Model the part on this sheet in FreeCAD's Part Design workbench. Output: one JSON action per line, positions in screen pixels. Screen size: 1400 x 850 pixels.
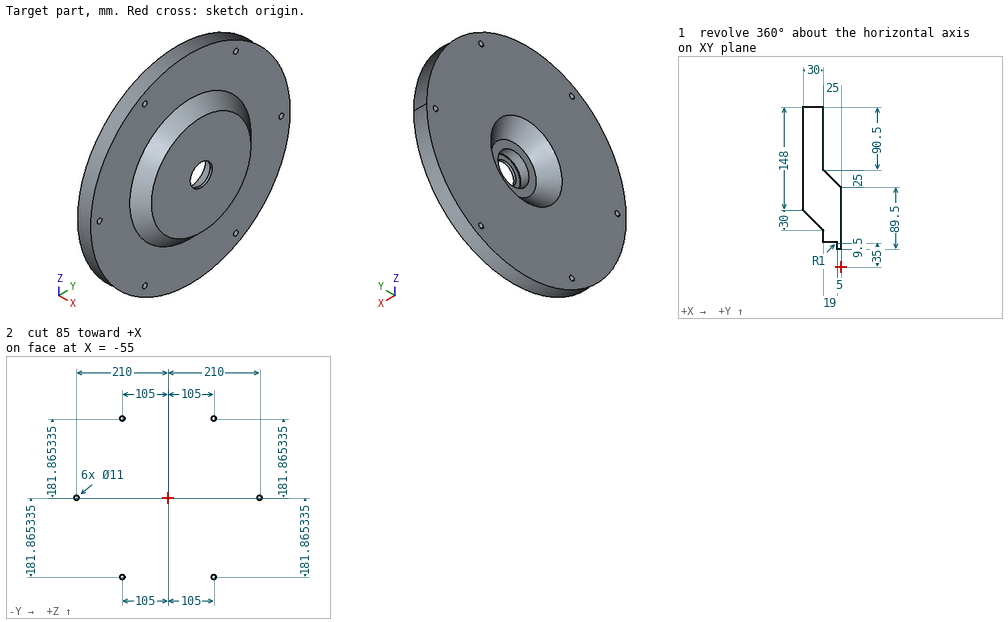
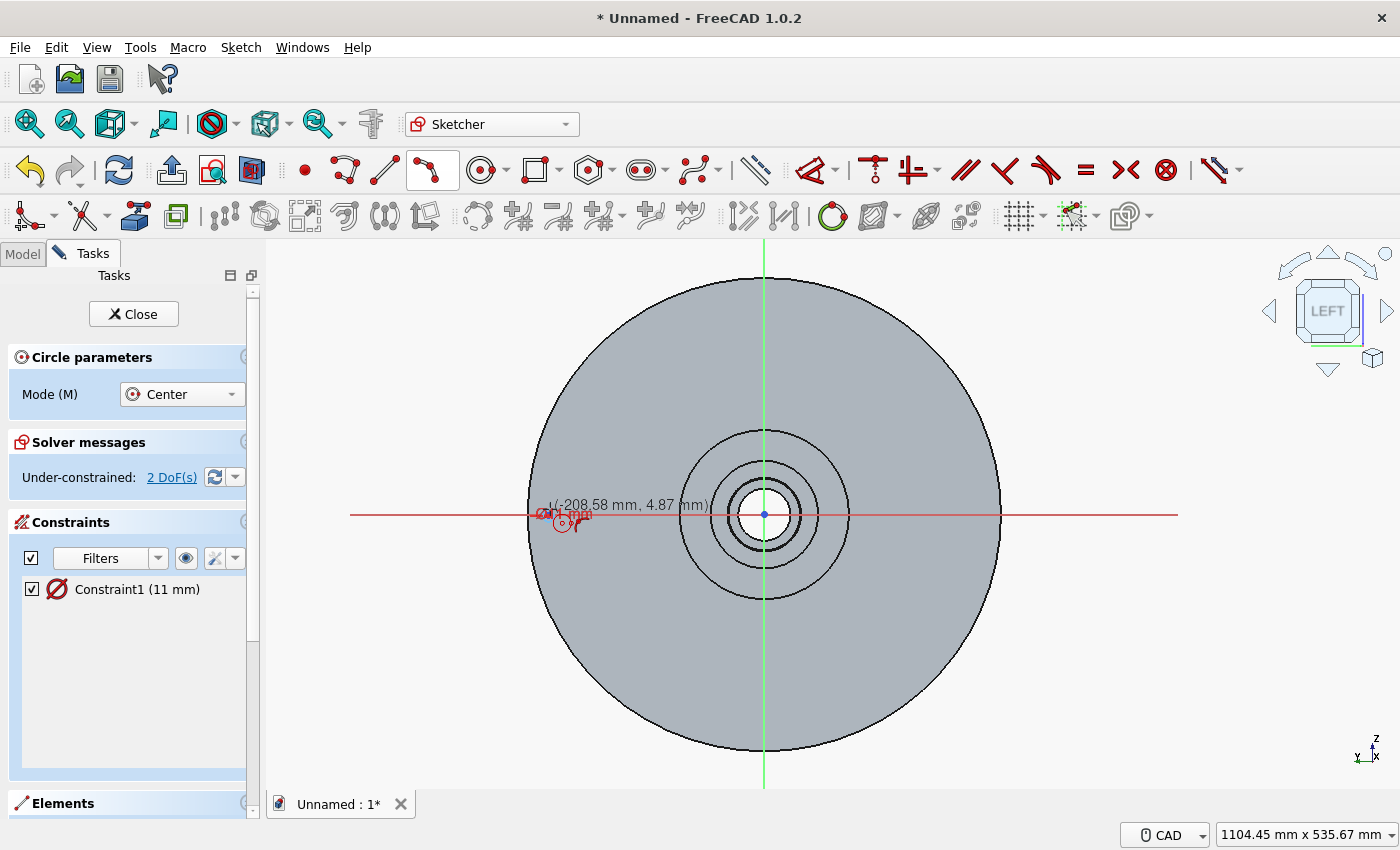
{"action": "scroll", "coordinate": [657, 328], "scroll_direction": "up", "scroll_amount": 7}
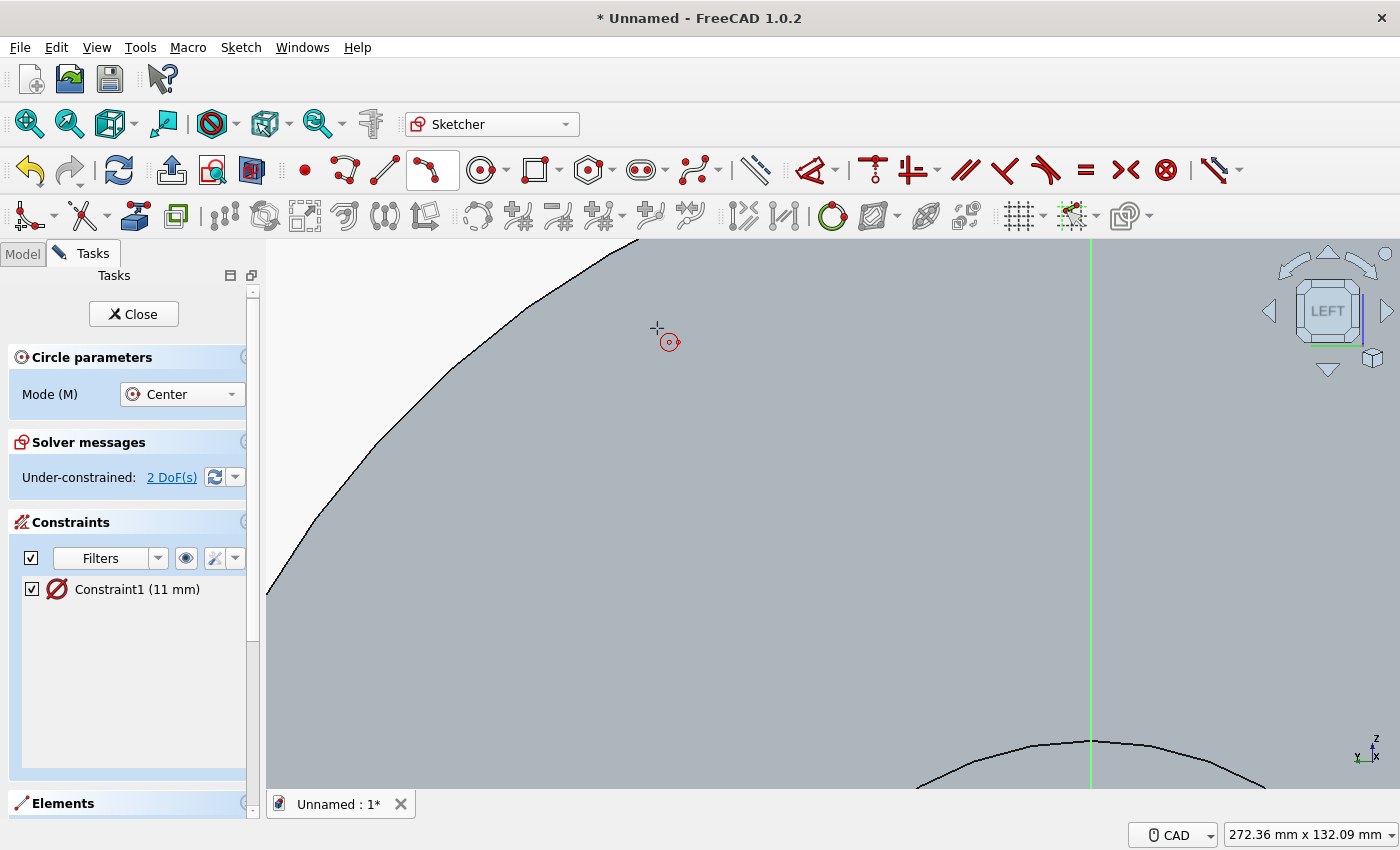
{"action": "scroll", "coordinate": [658, 327], "scroll_direction": "down", "scroll_amount": 7}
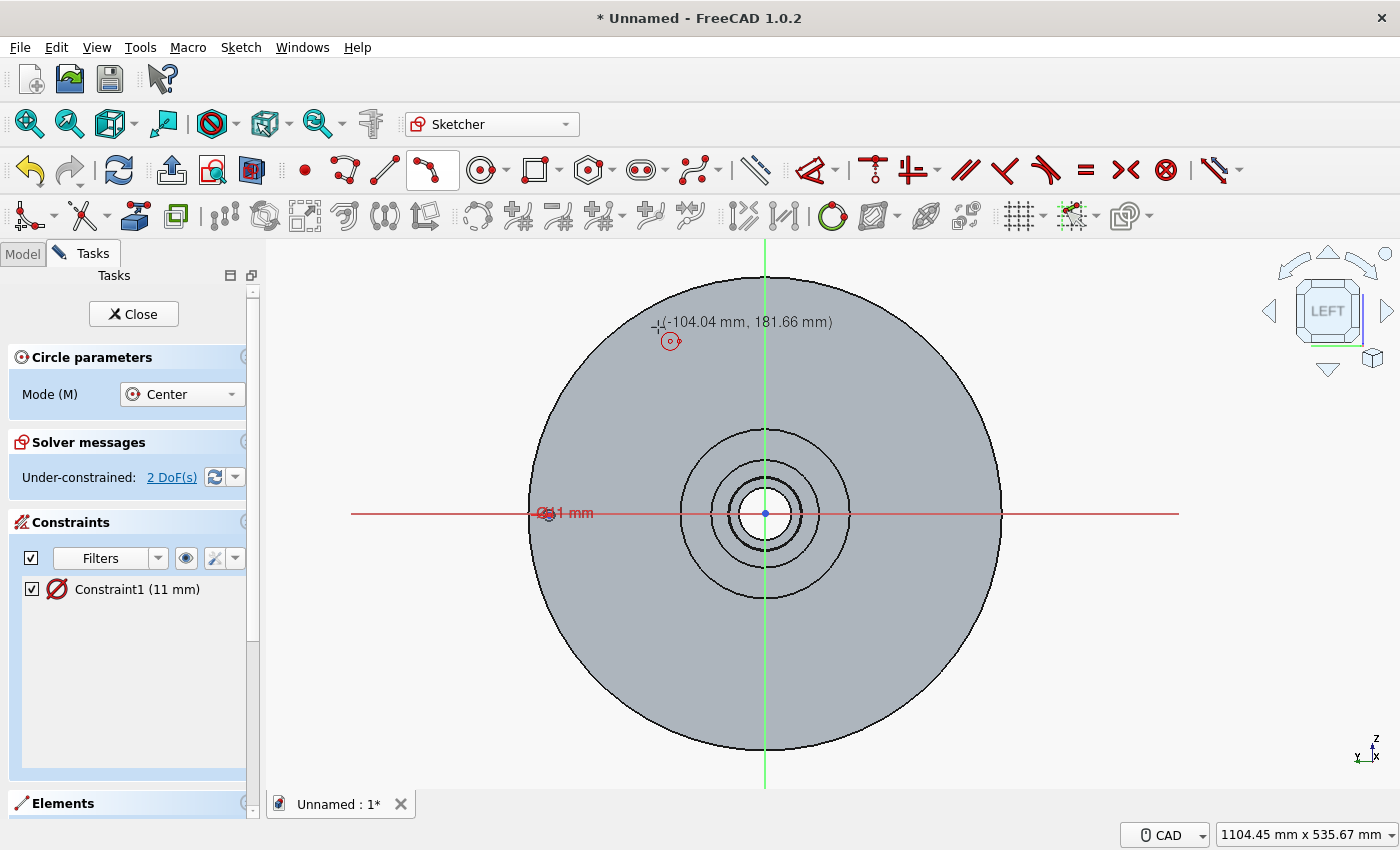
{"action": "left_click", "coordinate": [657, 327]}
{"action": "mouse_move", "coordinate": [661, 323]}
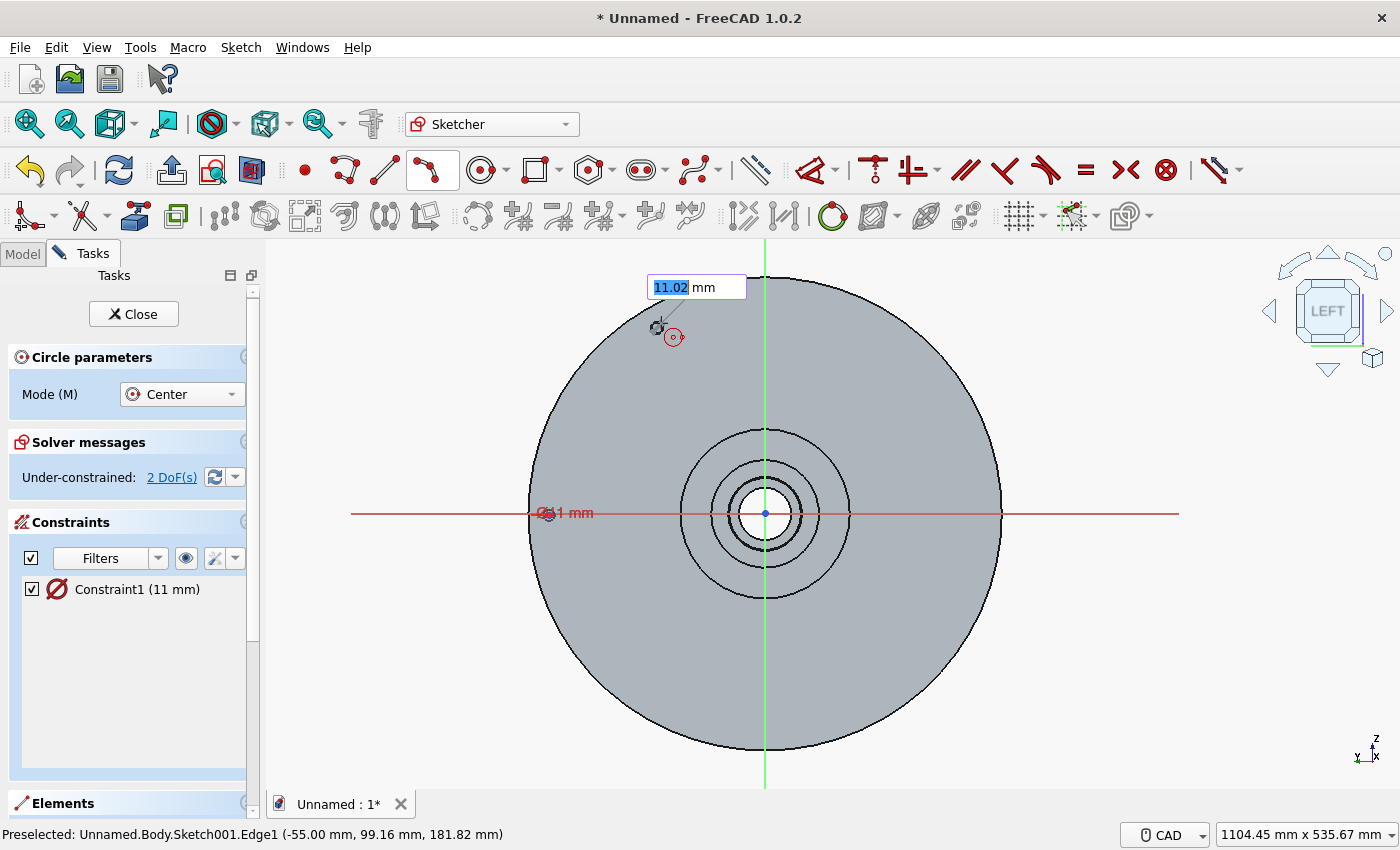
{"action": "type", "text": "11"}
{"action": "key", "text": "Return"}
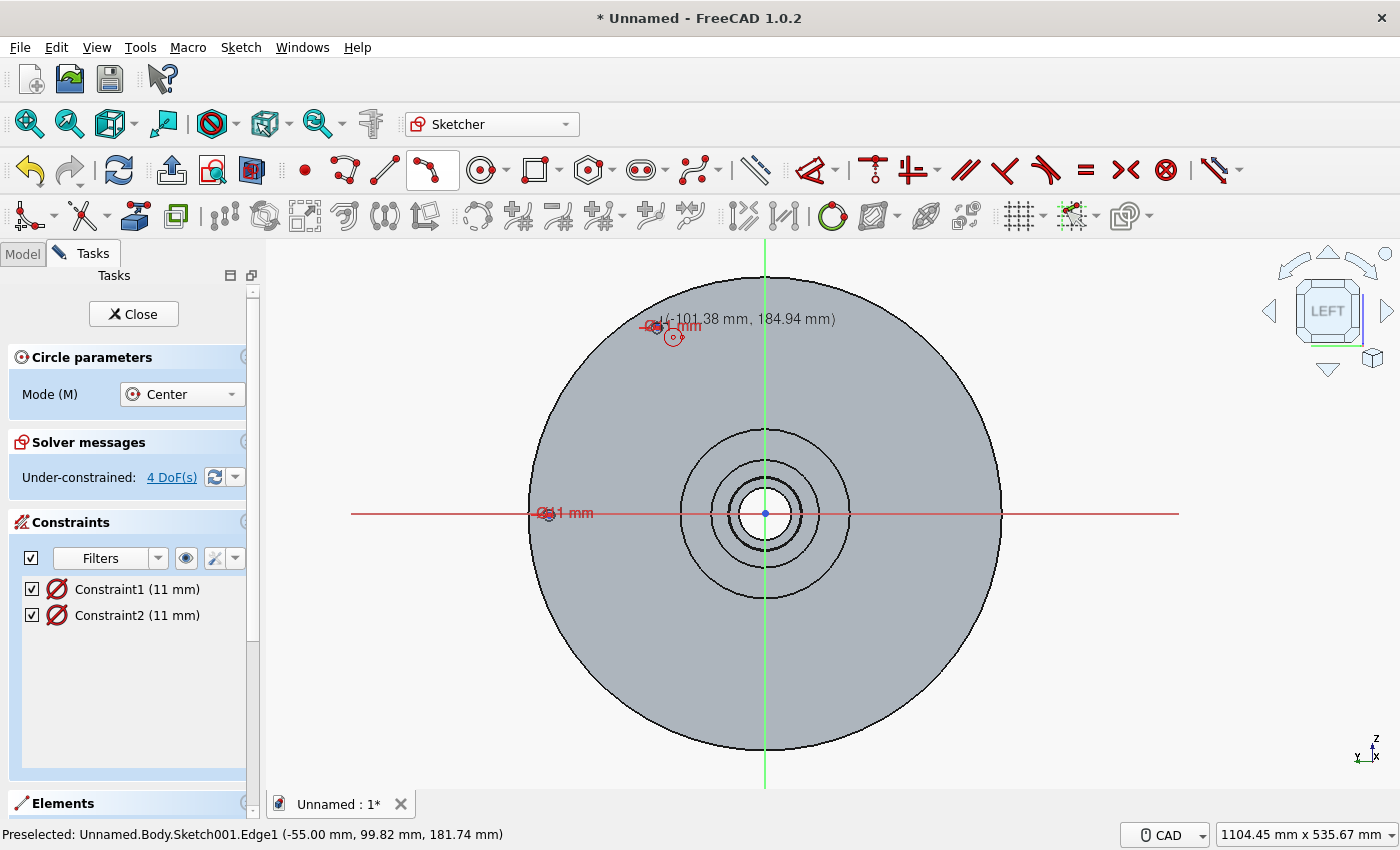
{"action": "scroll", "coordinate": [873, 327], "scroll_direction": "up", "scroll_amount": 7}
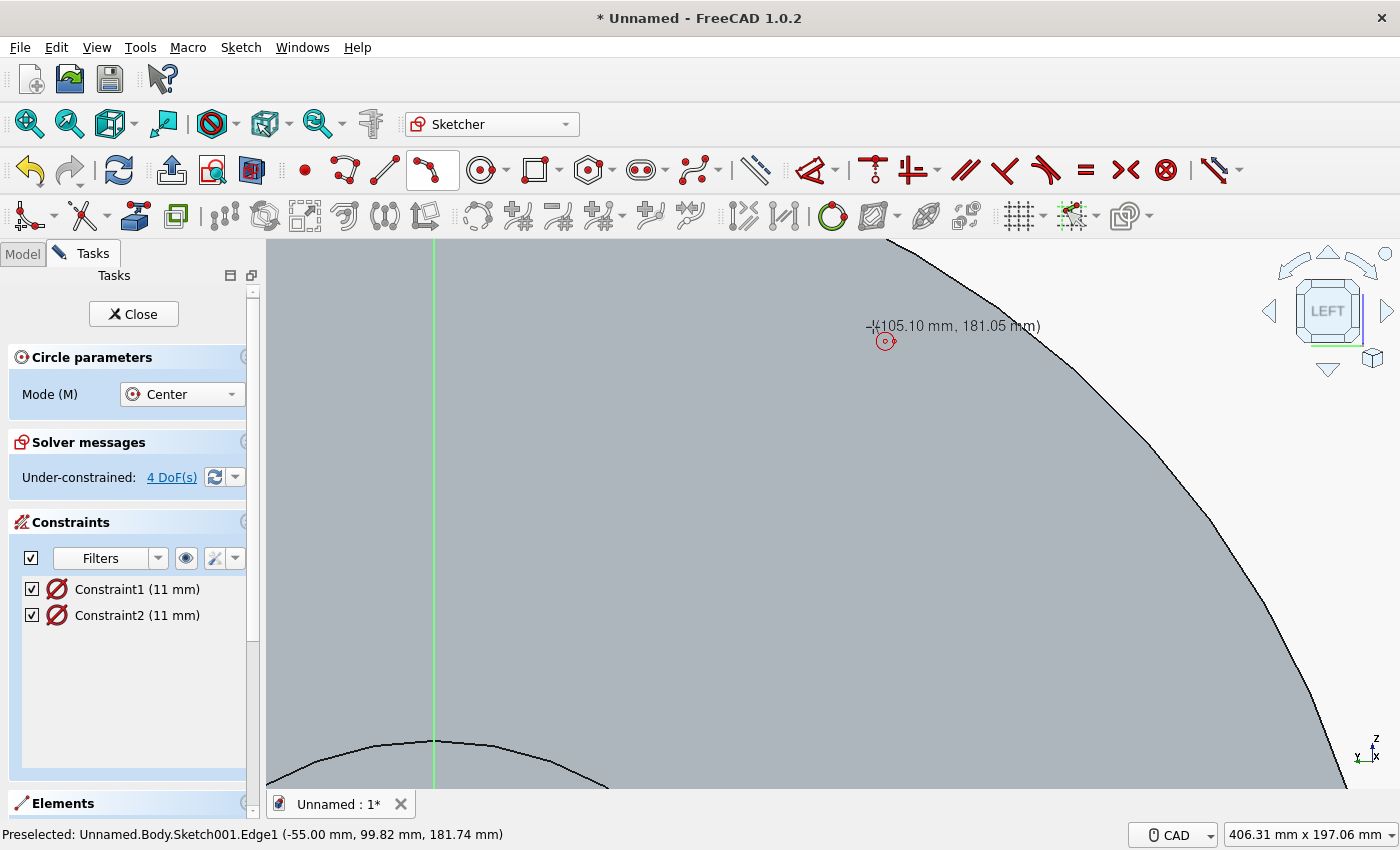
{"action": "scroll", "coordinate": [873, 327], "scroll_direction": "down", "scroll_amount": 7}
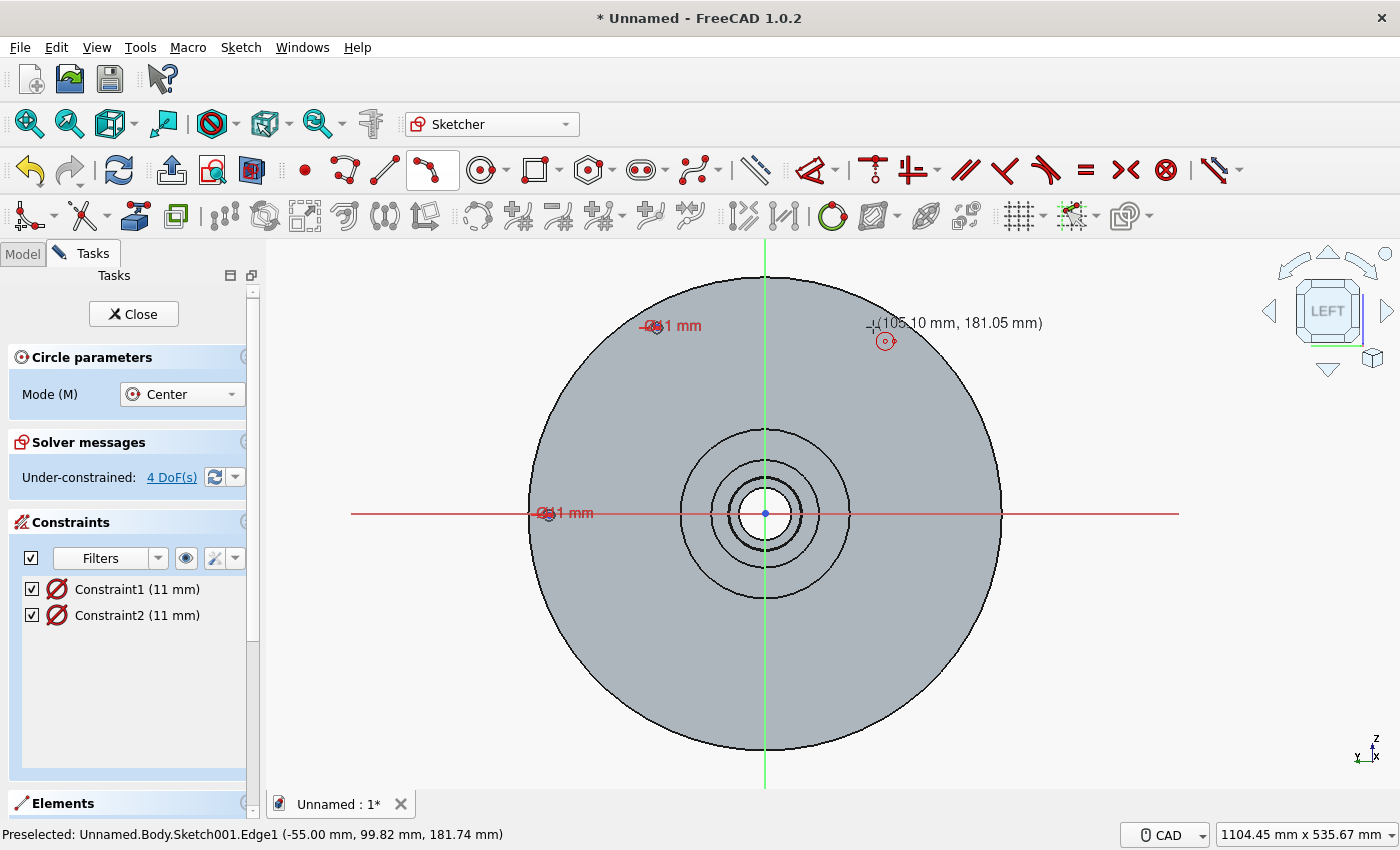
{"action": "left_click", "coordinate": [873, 327]}
{"action": "mouse_move", "coordinate": [877, 323]}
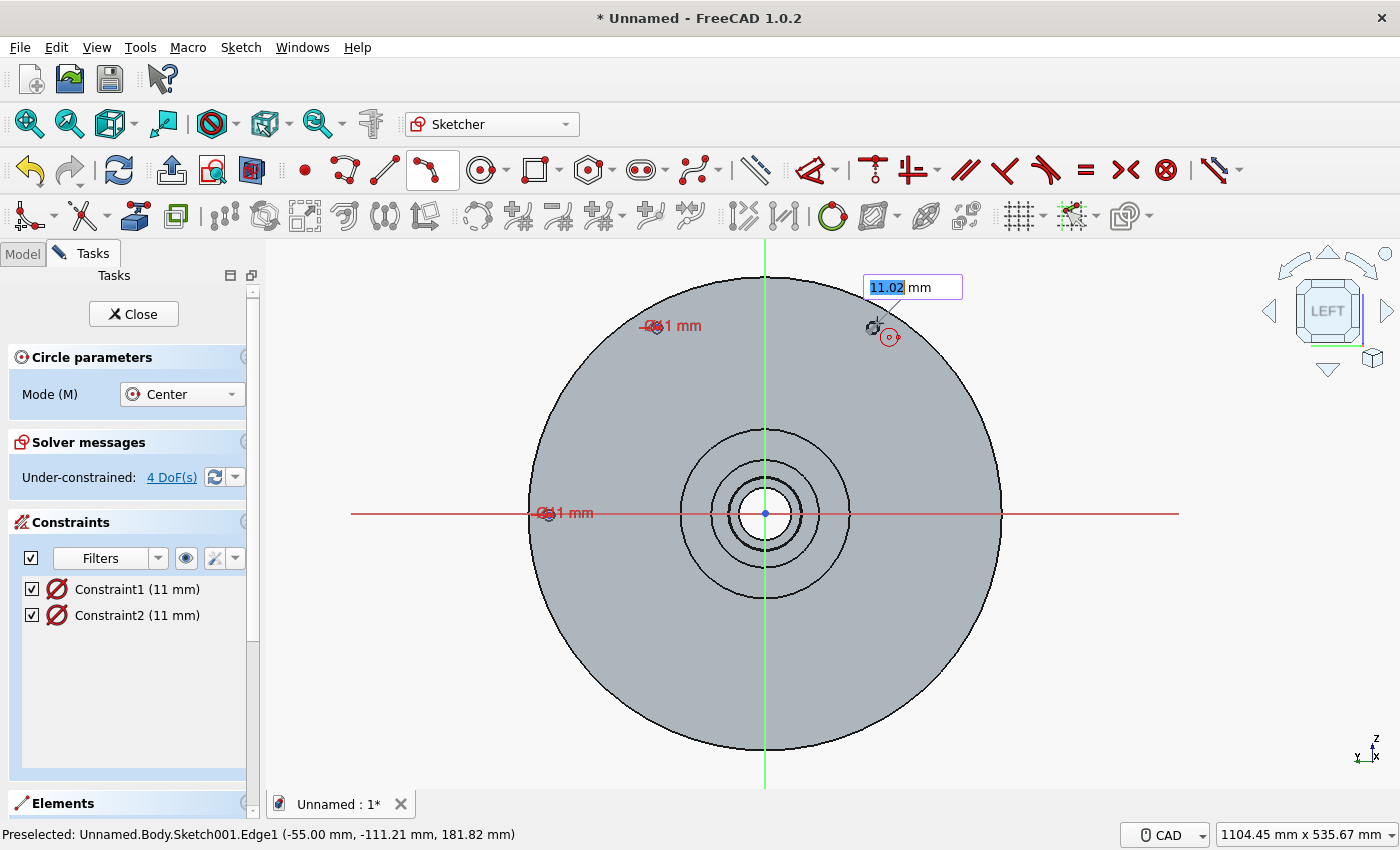
{"action": "type", "text": "11"}
{"action": "key", "text": "Return"}